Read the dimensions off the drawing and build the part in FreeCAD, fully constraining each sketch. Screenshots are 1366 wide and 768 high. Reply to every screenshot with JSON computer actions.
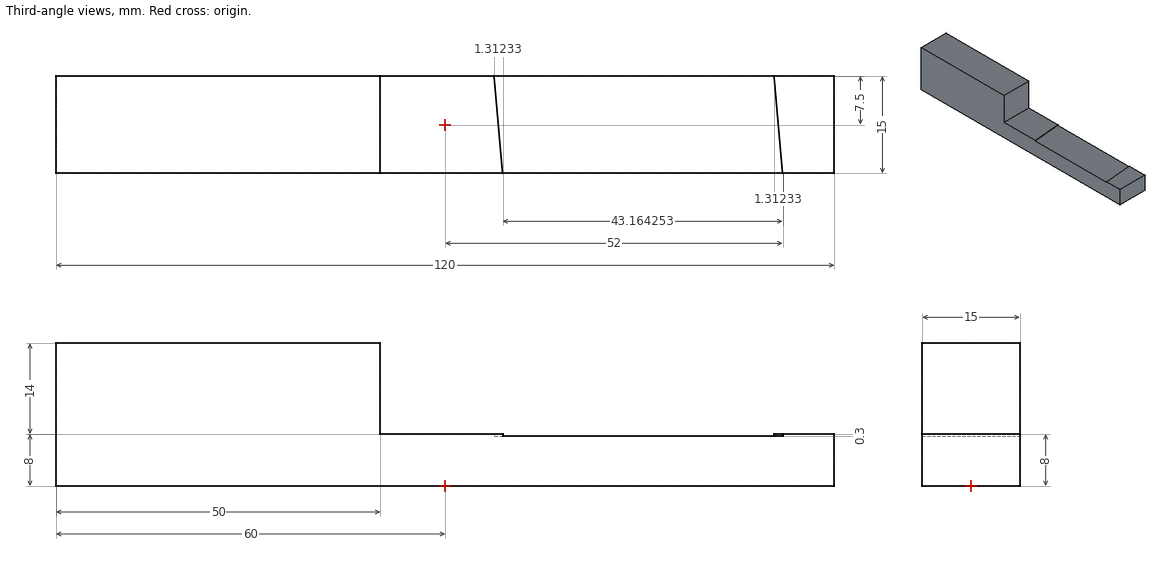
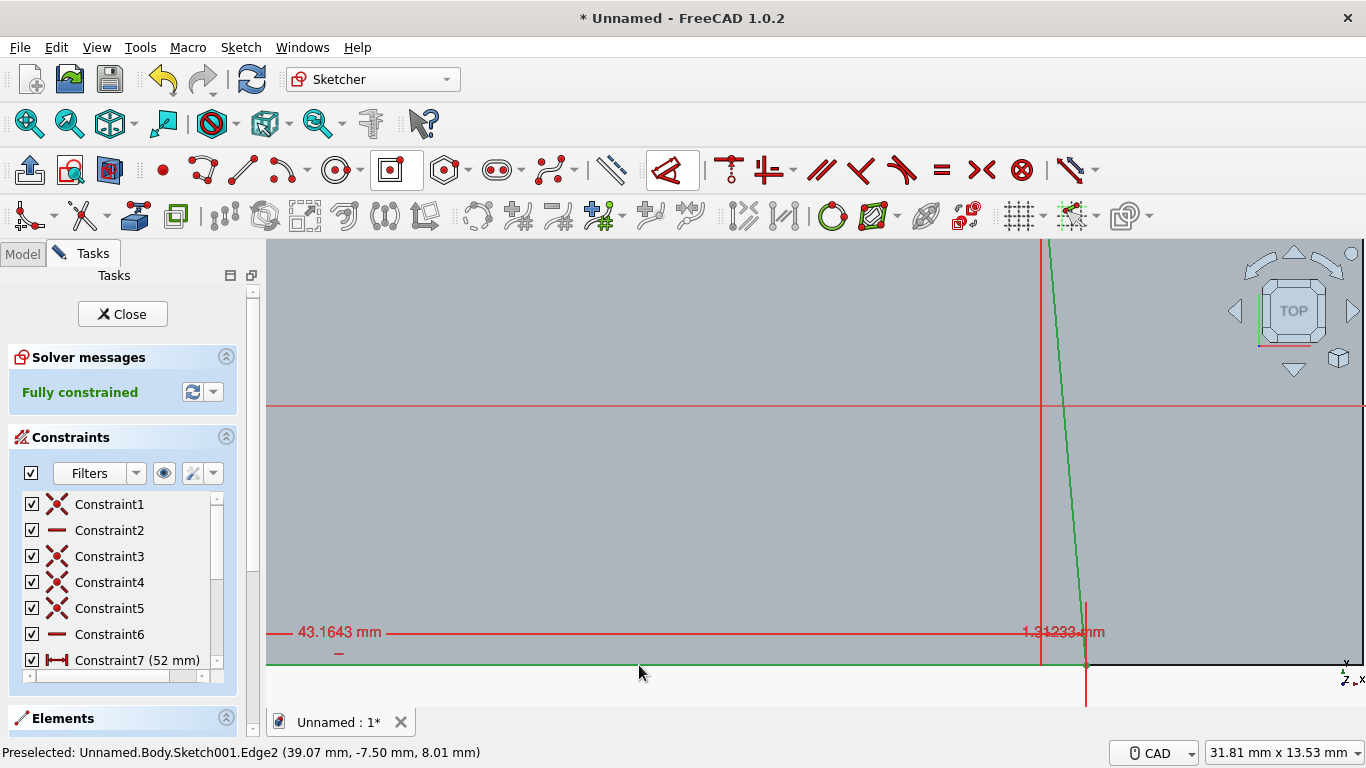
{"action": "left_click", "coordinate": [123, 314]}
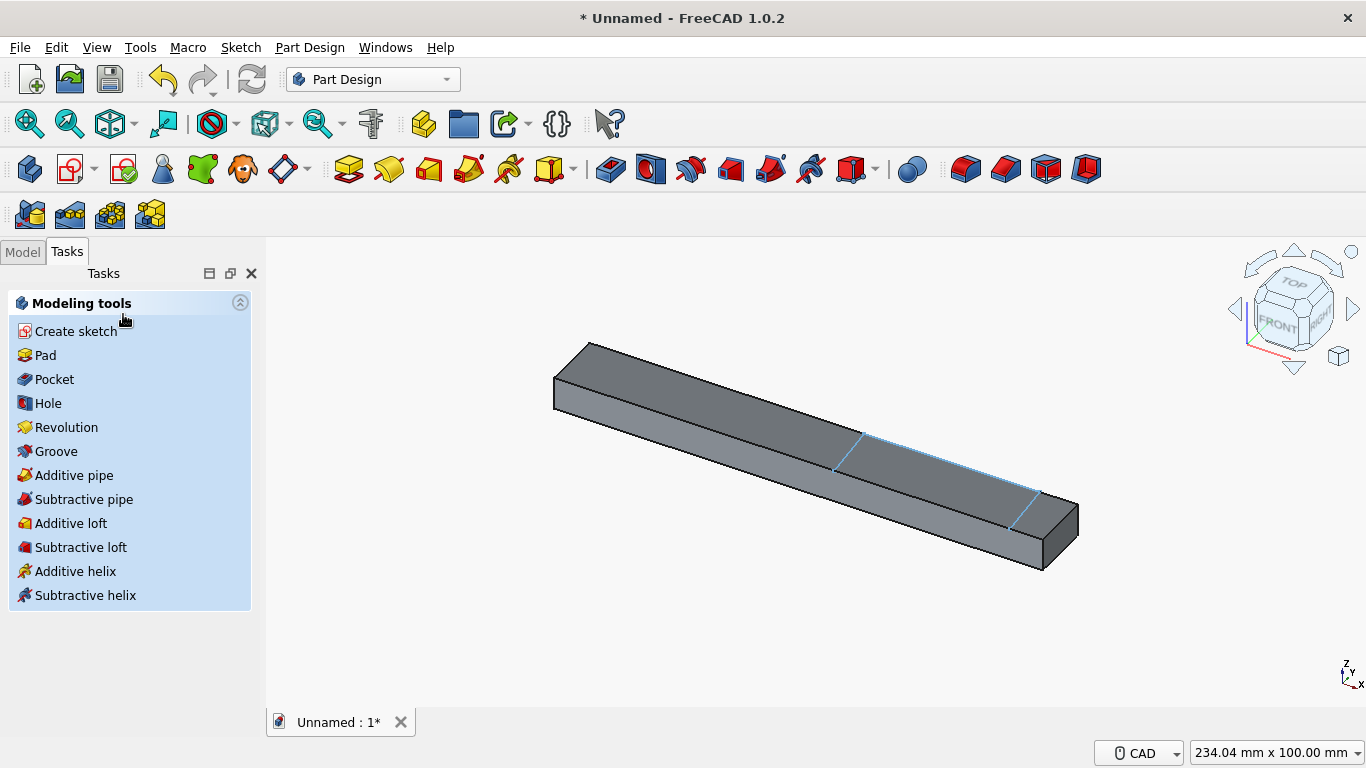
{"action": "left_click", "coordinate": [612, 170]}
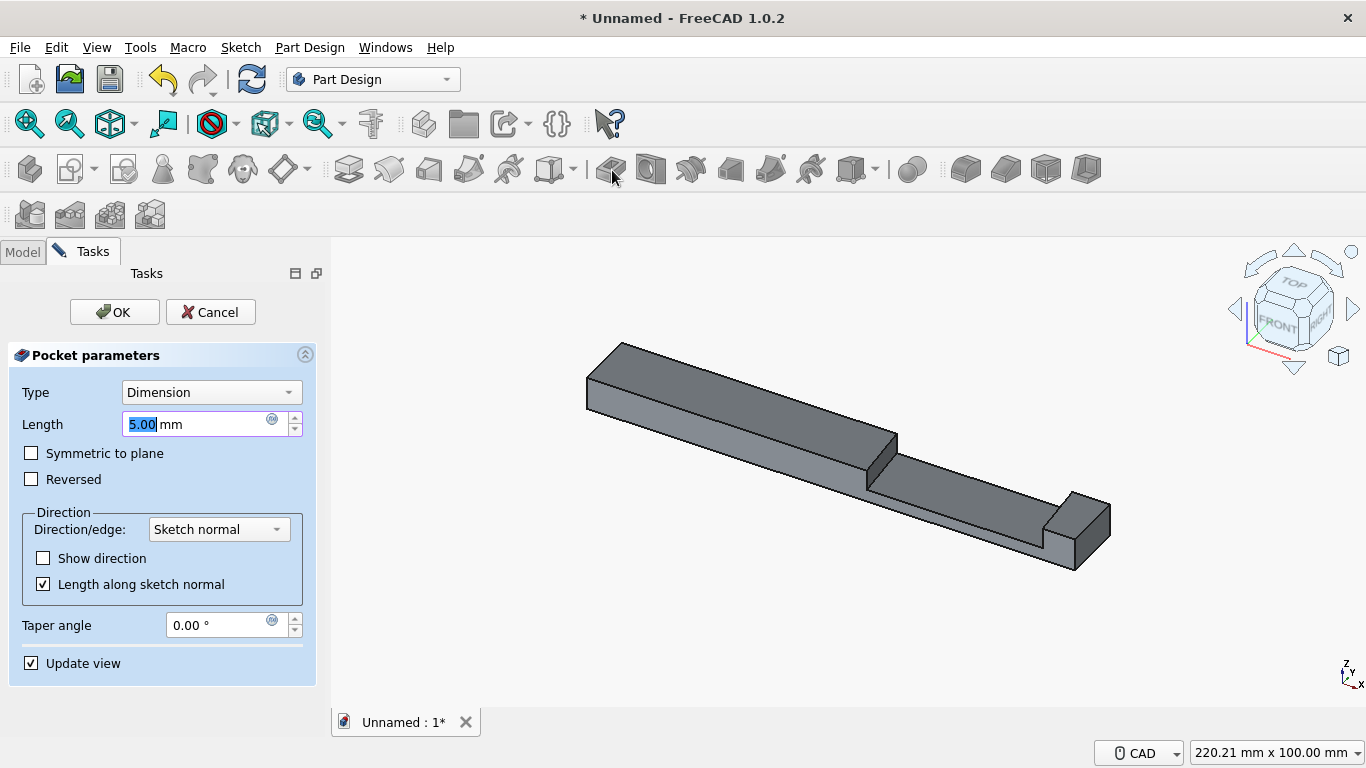
{"action": "type", "text": "0.3"}
{"action": "key", "text": "Tab"}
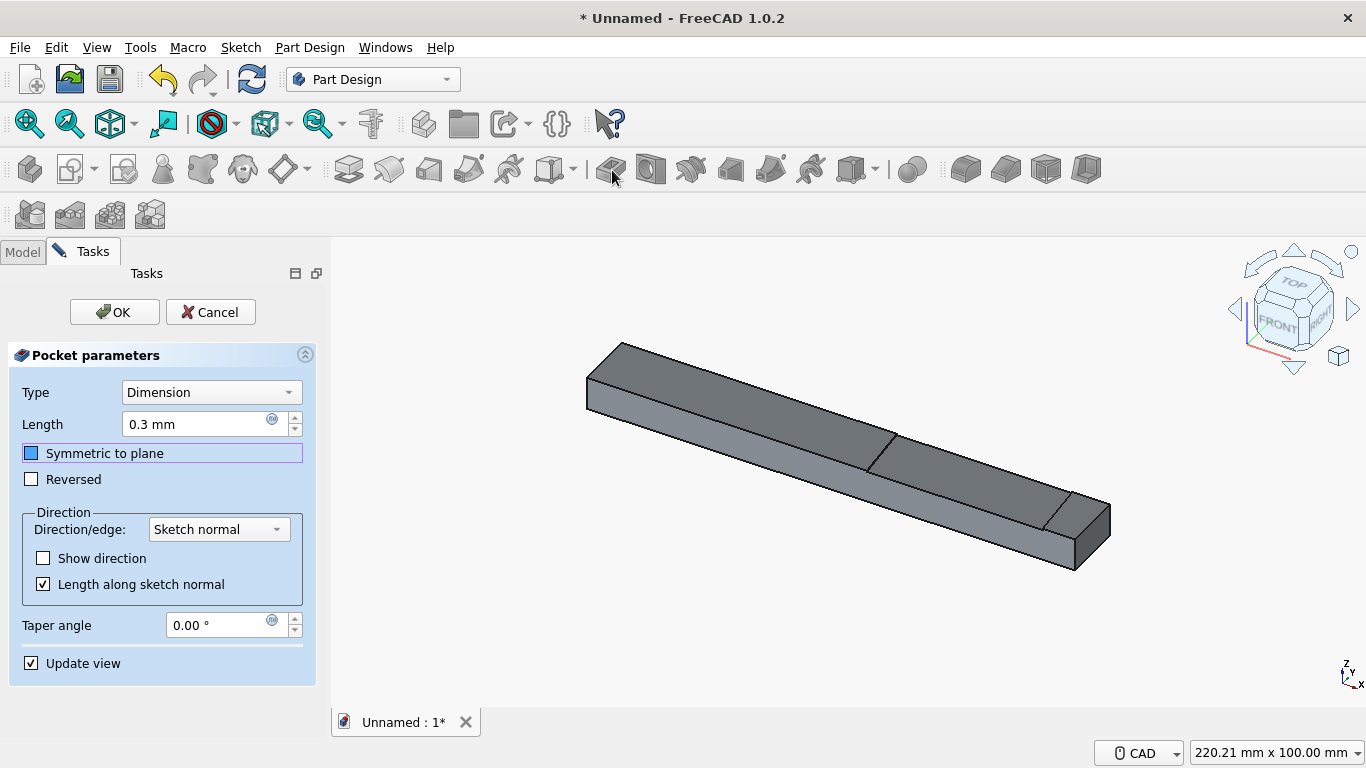
{"action": "left_click", "coordinate": [115, 312]}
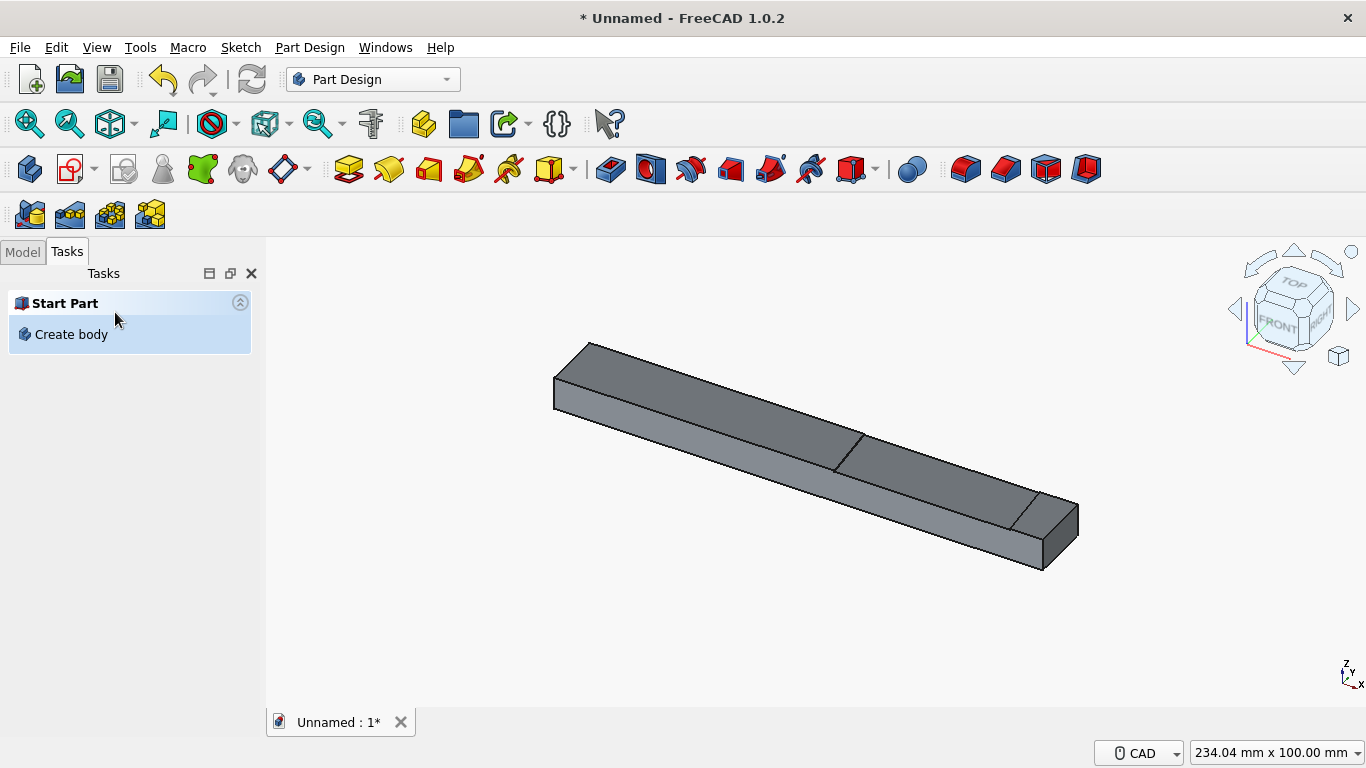
{"action": "left_click", "coordinate": [798, 473]}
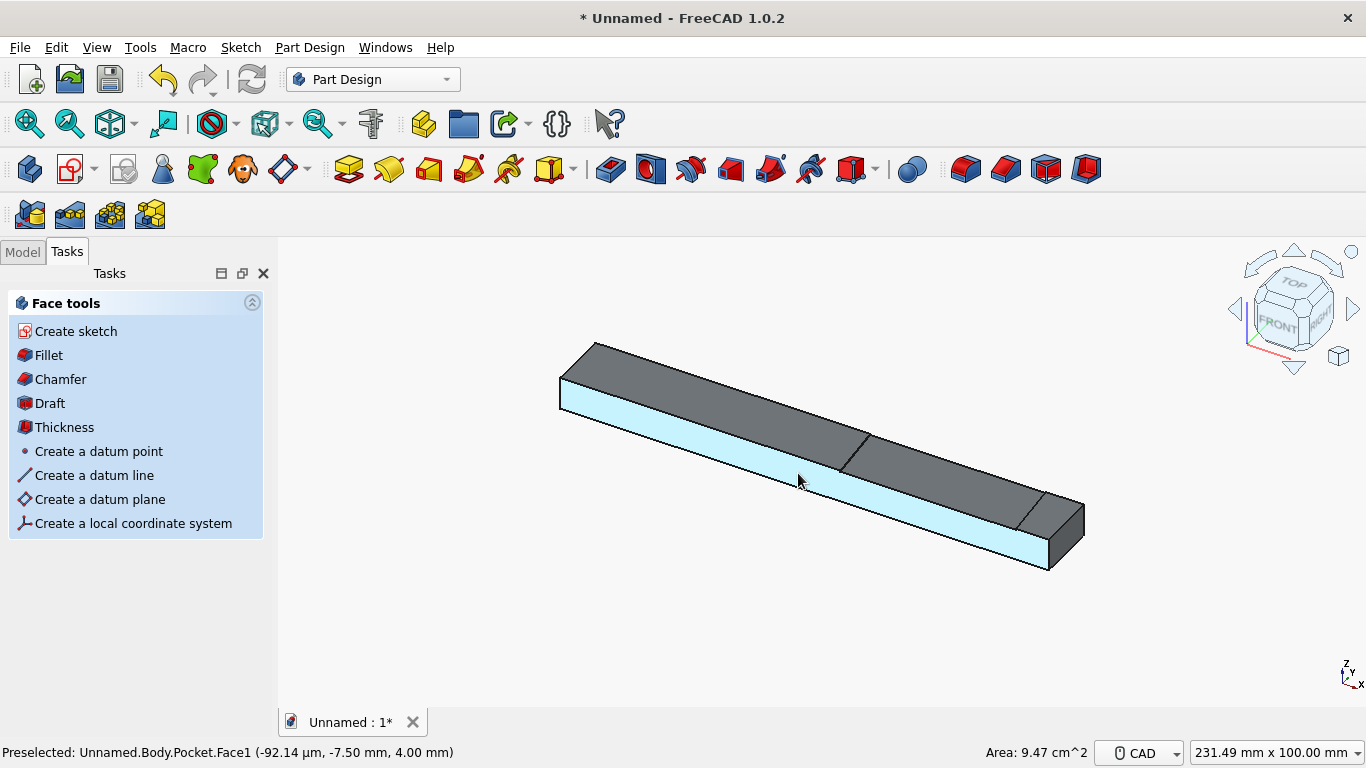
{"action": "left_click", "coordinate": [70, 170]}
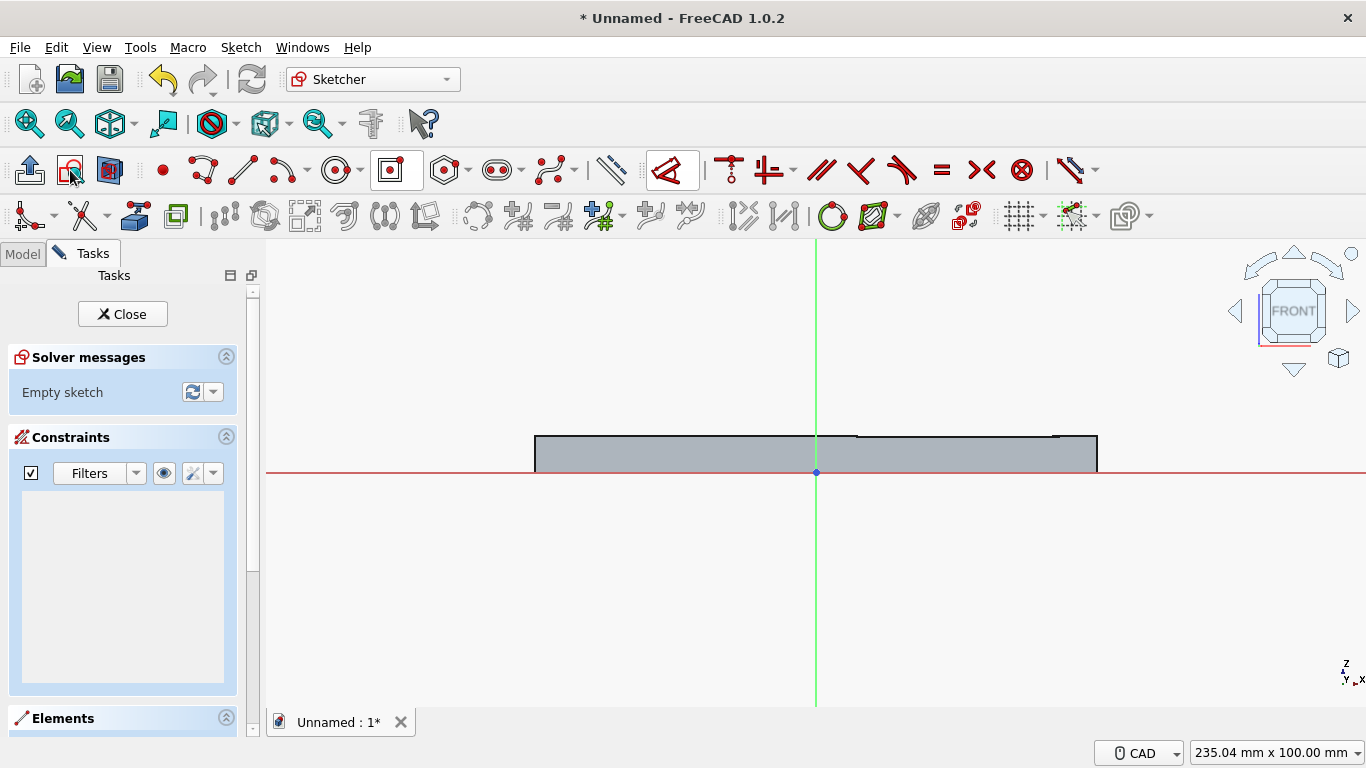
{"action": "scroll", "coordinate": [617, 380], "scroll_direction": "up", "scroll_amount": 4}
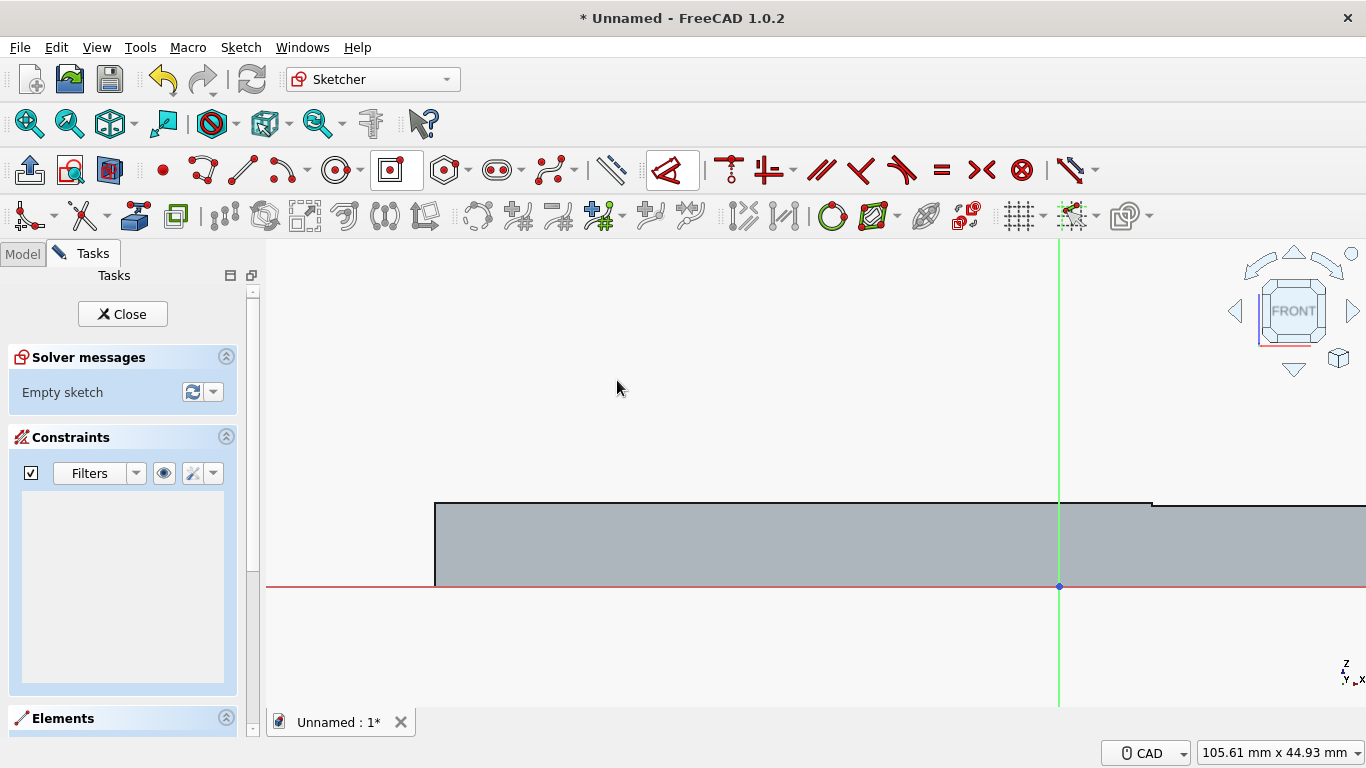
{"action": "left_click", "coordinate": [418, 170]}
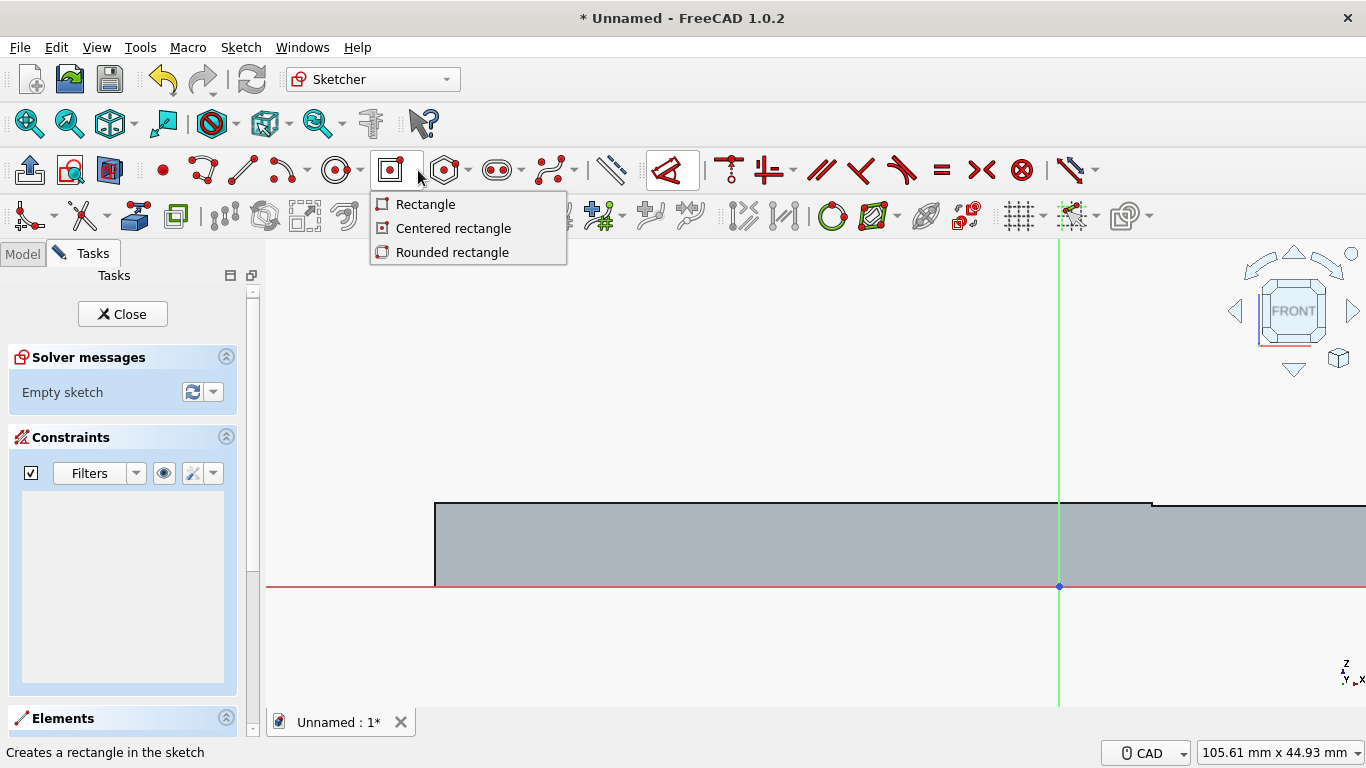
{"action": "left_click", "coordinate": [468, 204]}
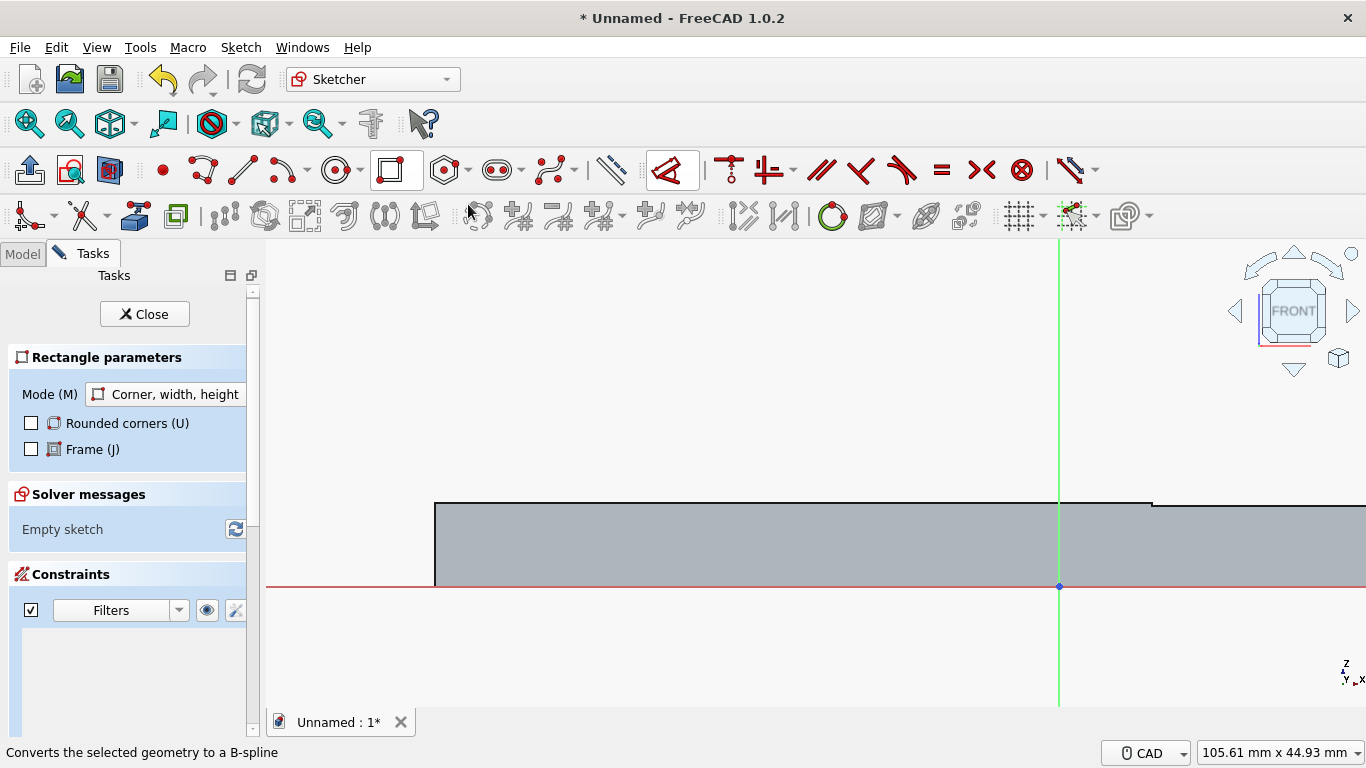
{"action": "left_click", "coordinate": [435, 357]}
{"action": "mouse_move", "coordinate": [955, 503]}